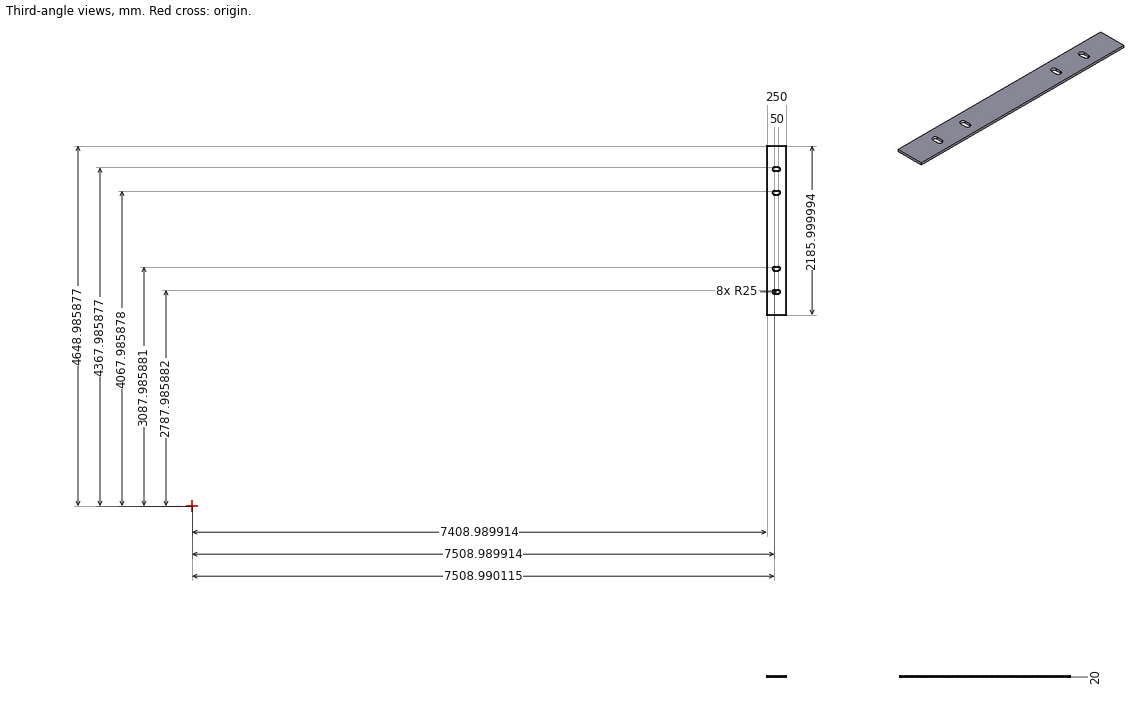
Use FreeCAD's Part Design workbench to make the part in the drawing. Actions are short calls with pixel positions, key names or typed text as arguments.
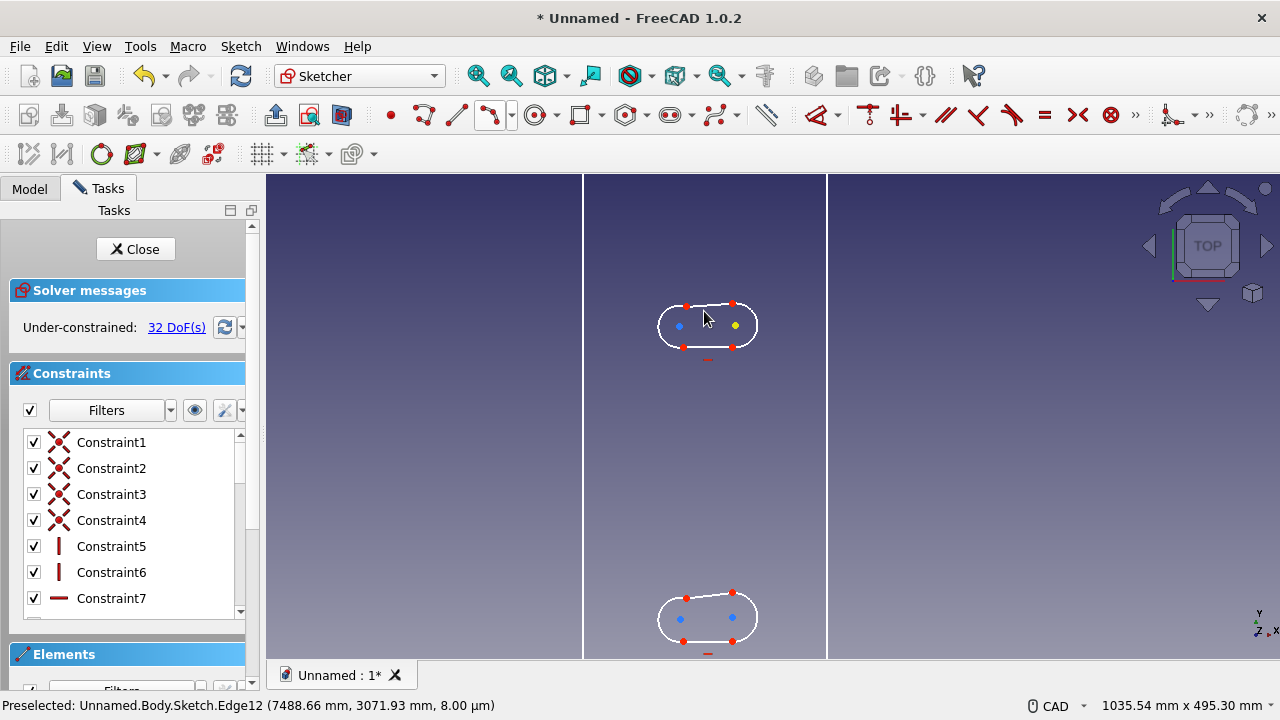
click(700, 306)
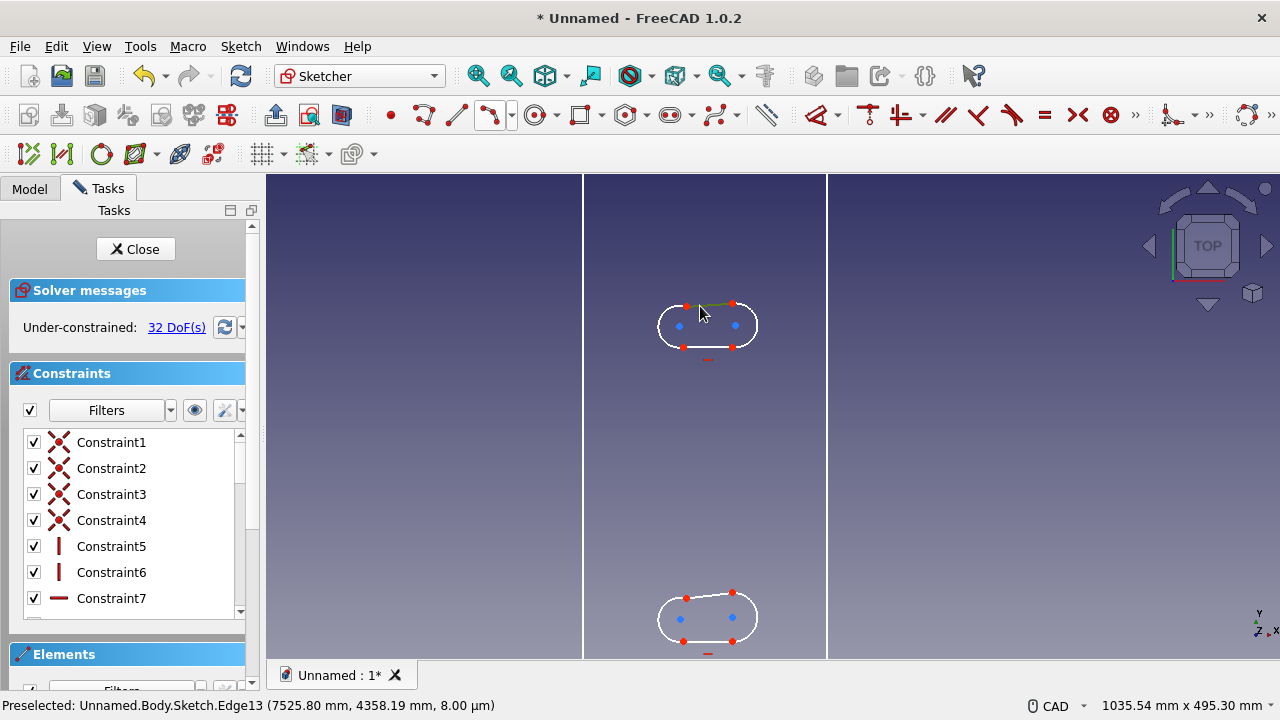
click(753, 339)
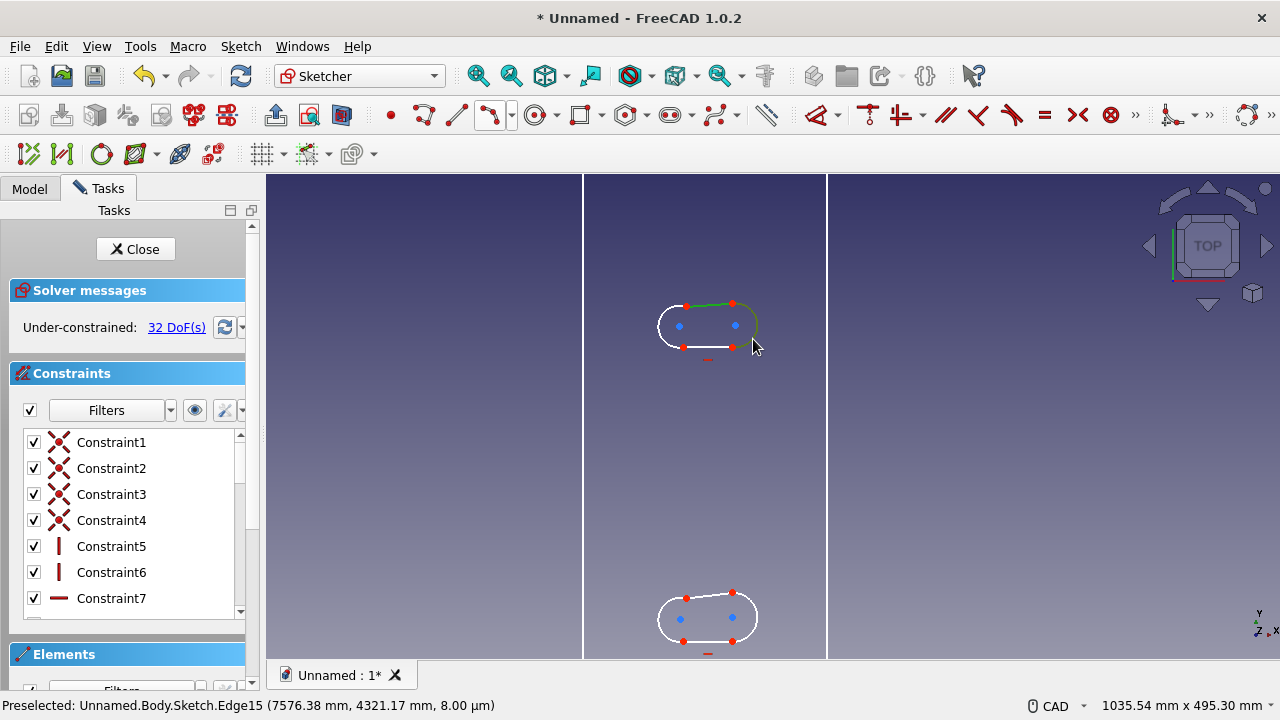
click(1012, 116)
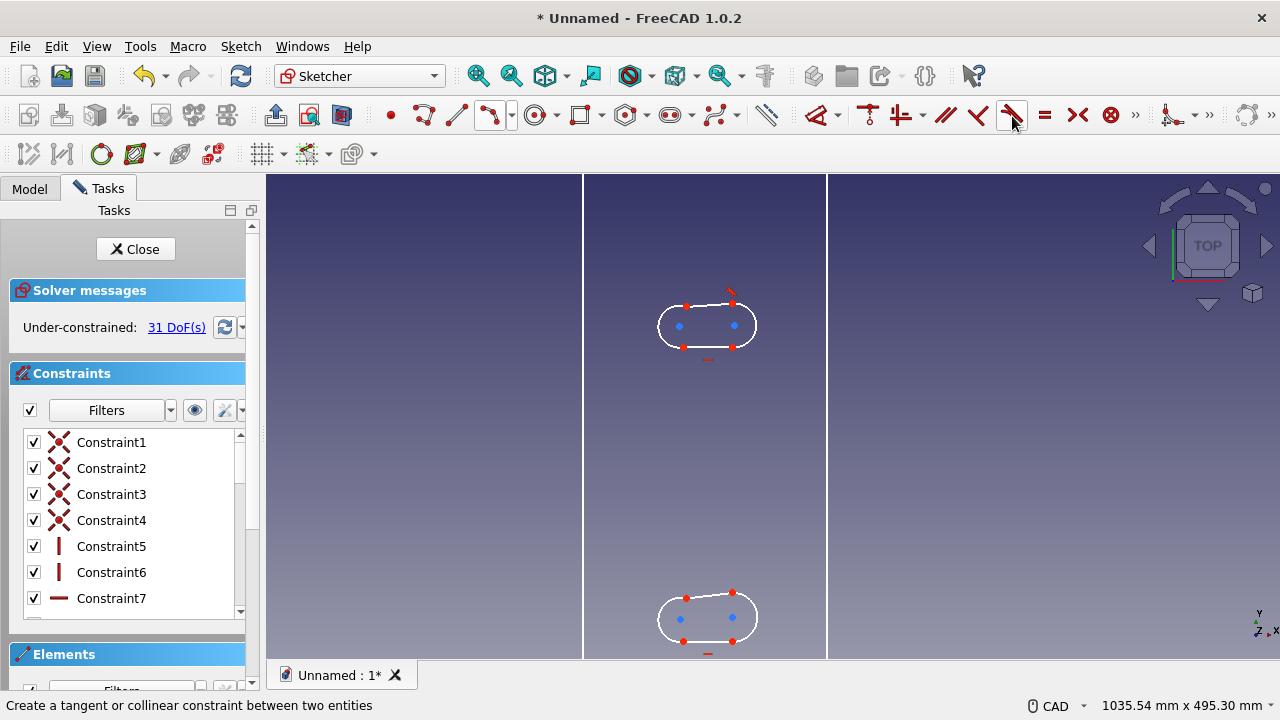
click(700, 306)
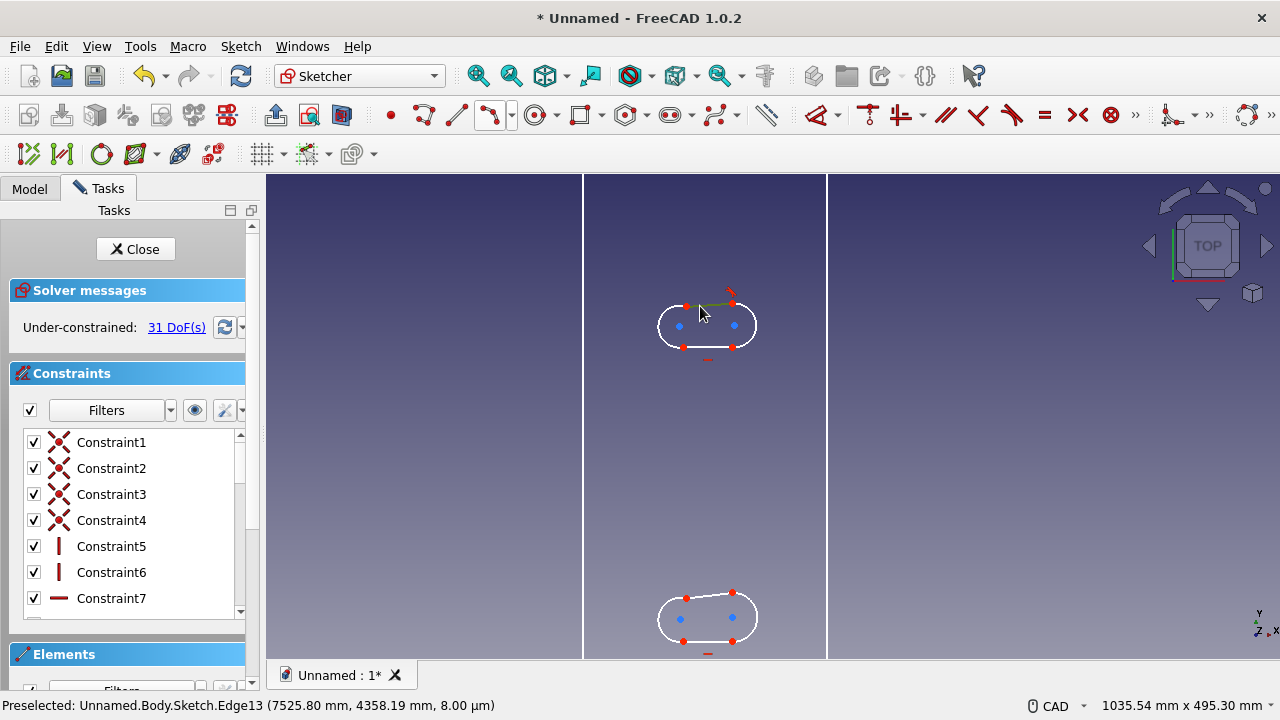
click(665, 312)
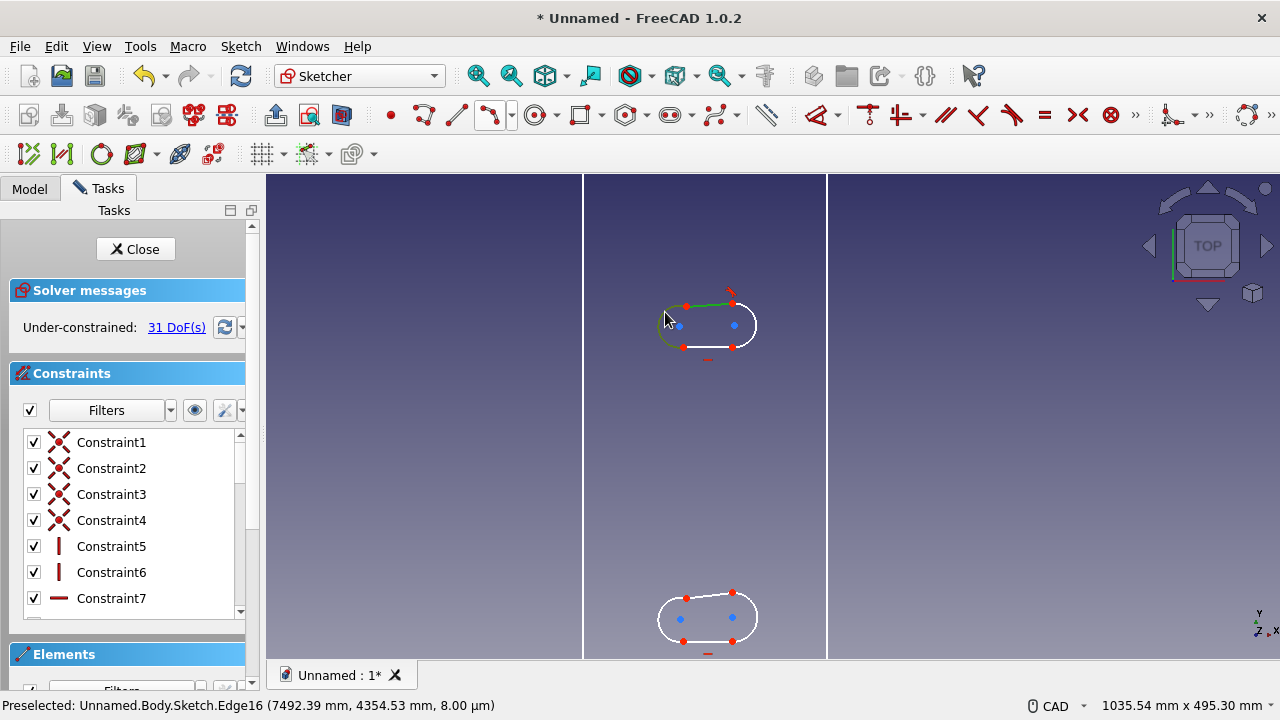
click(1012, 116)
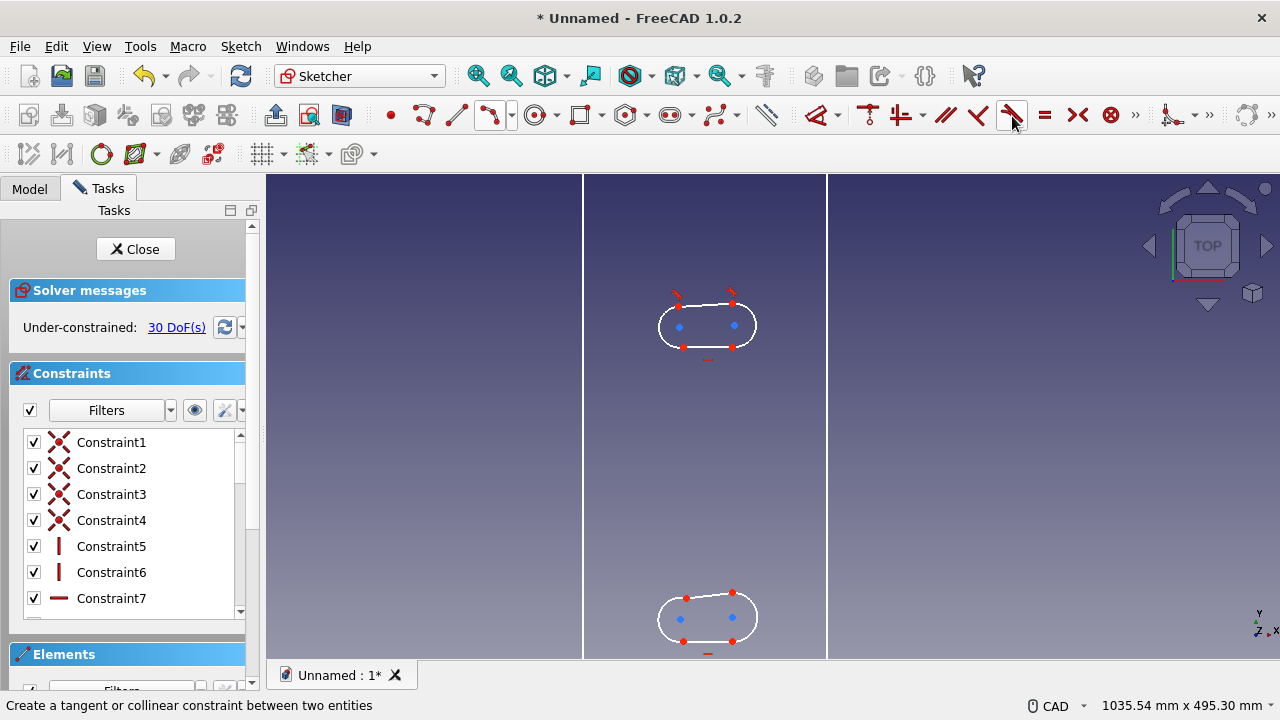
click(718, 347)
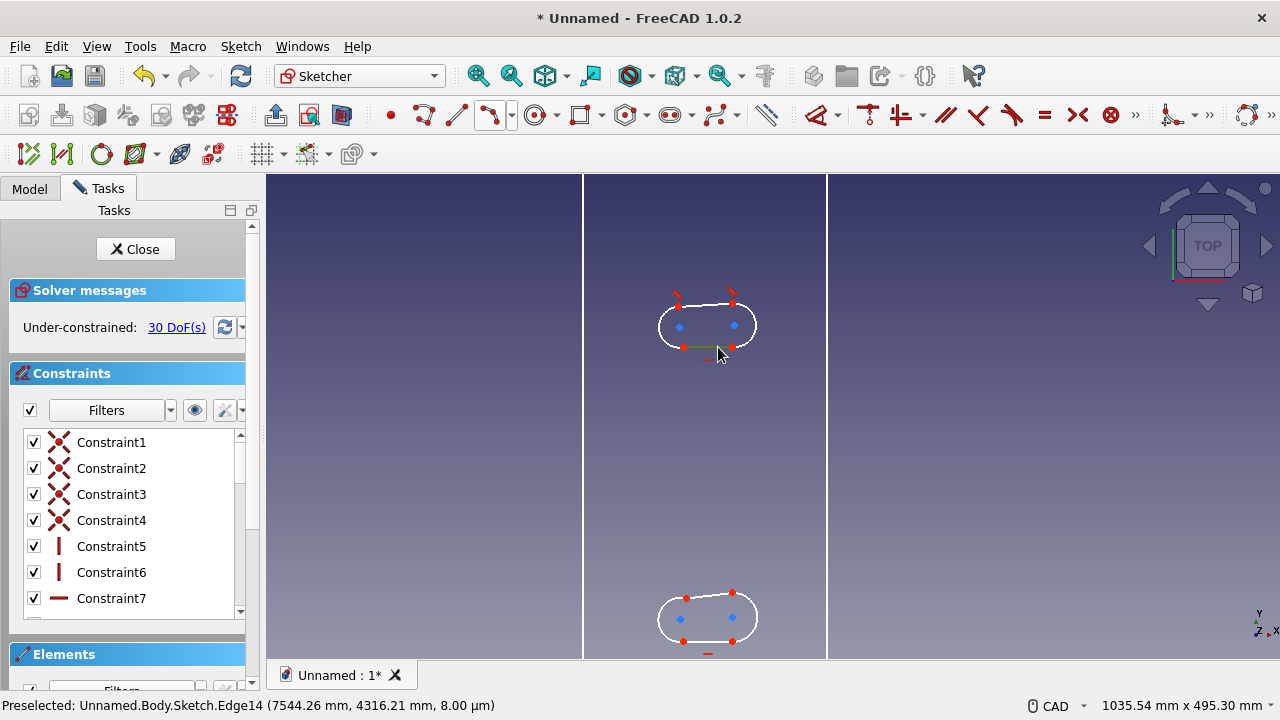
click(751, 339)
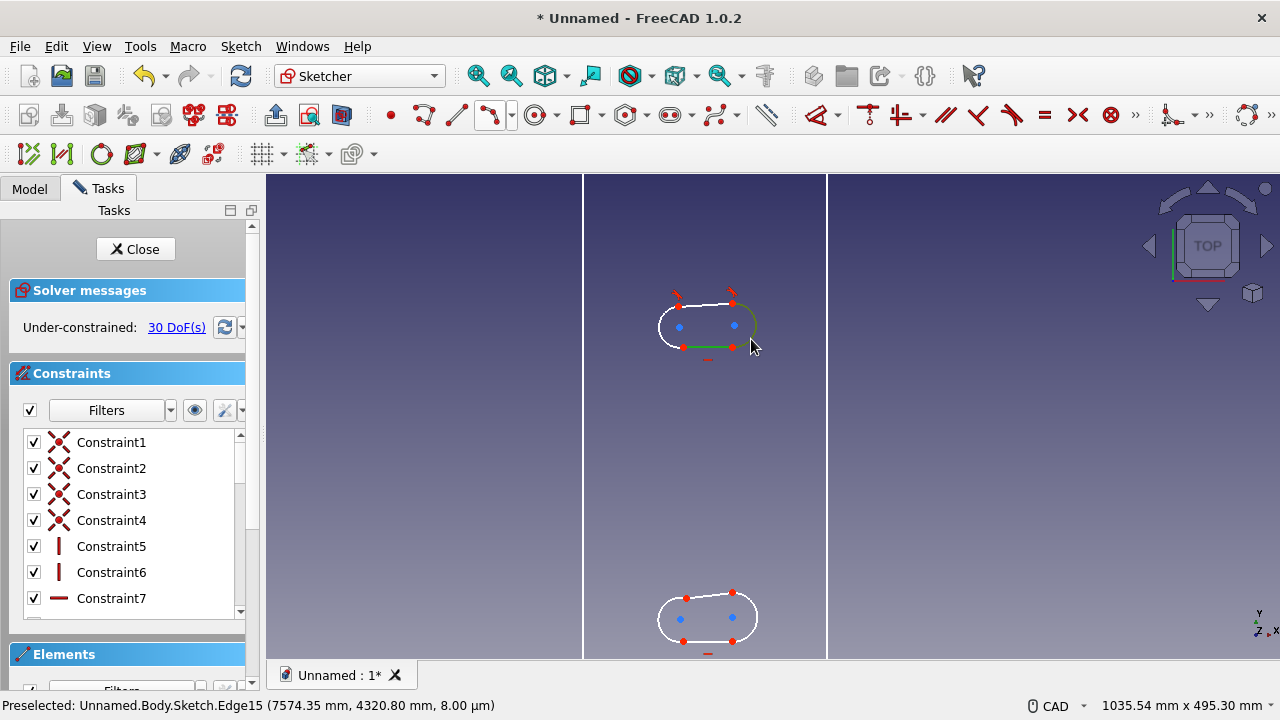
key(t)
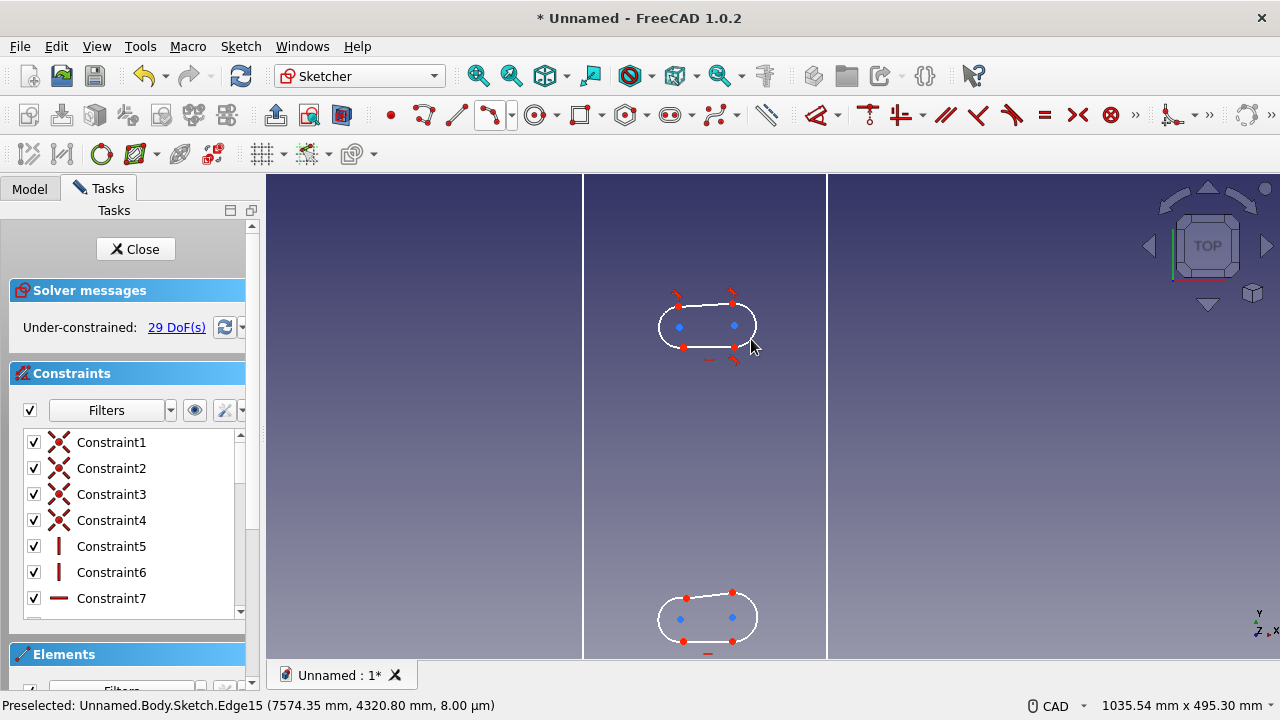
click(719, 347)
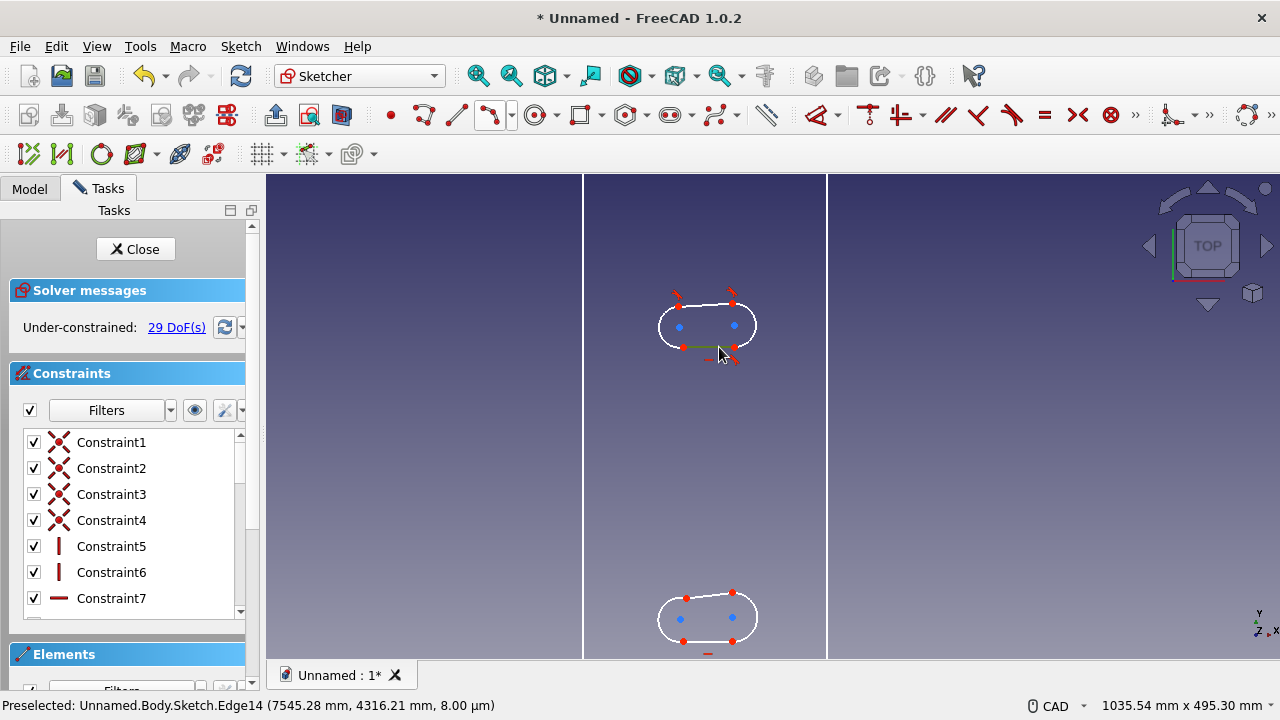
click(662, 317)